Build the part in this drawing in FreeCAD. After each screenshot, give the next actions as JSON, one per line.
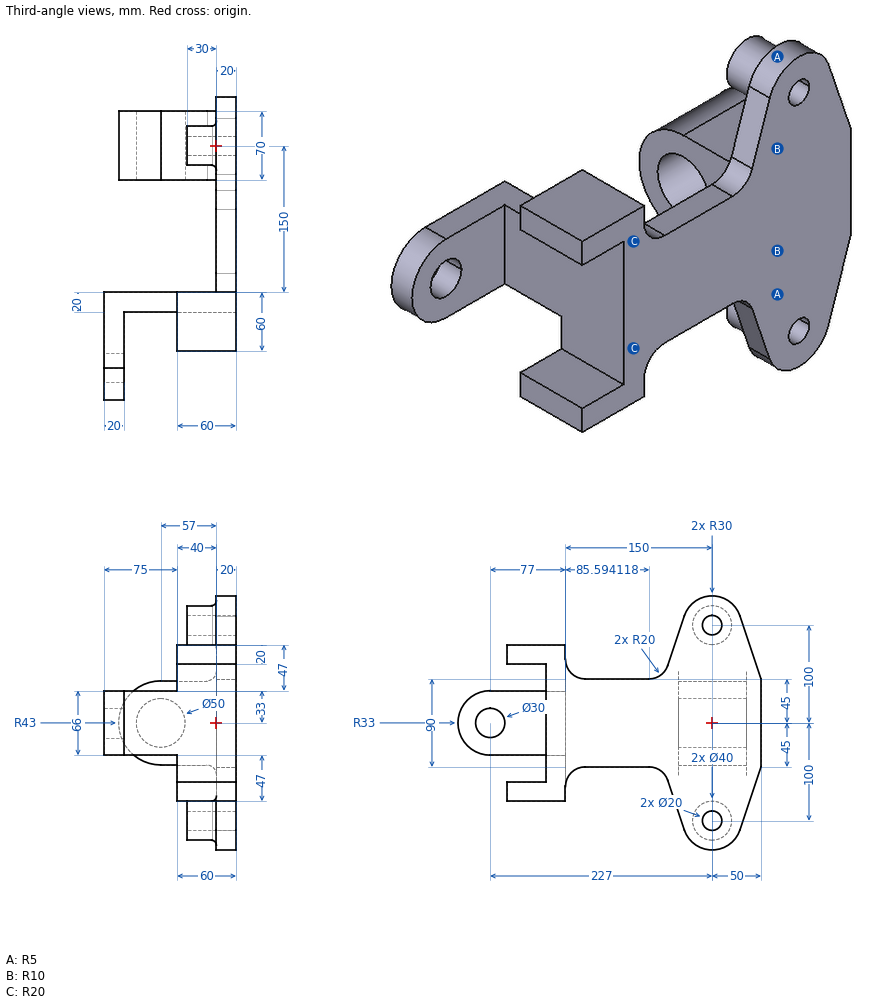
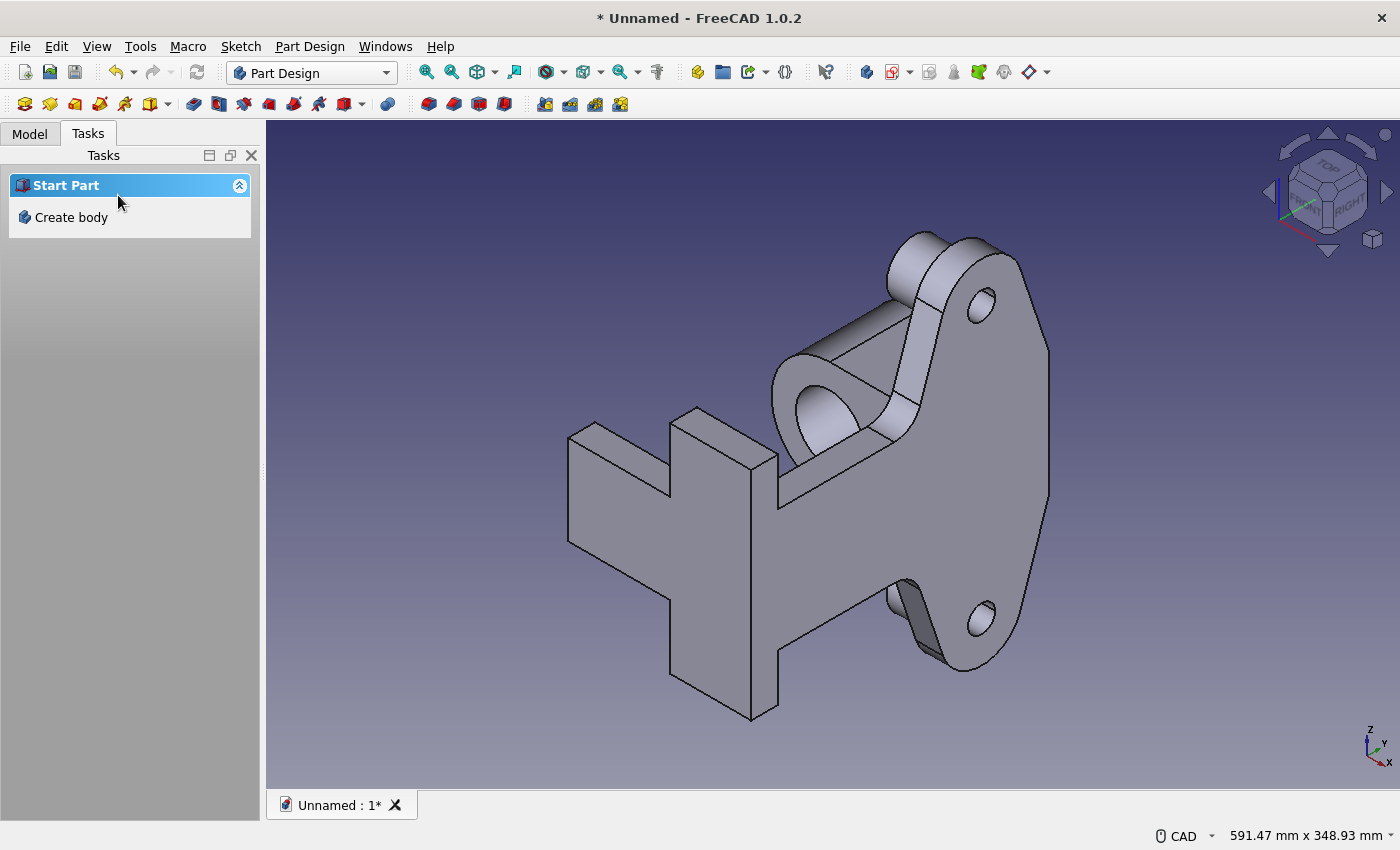
{"action": "key", "text": "v f"}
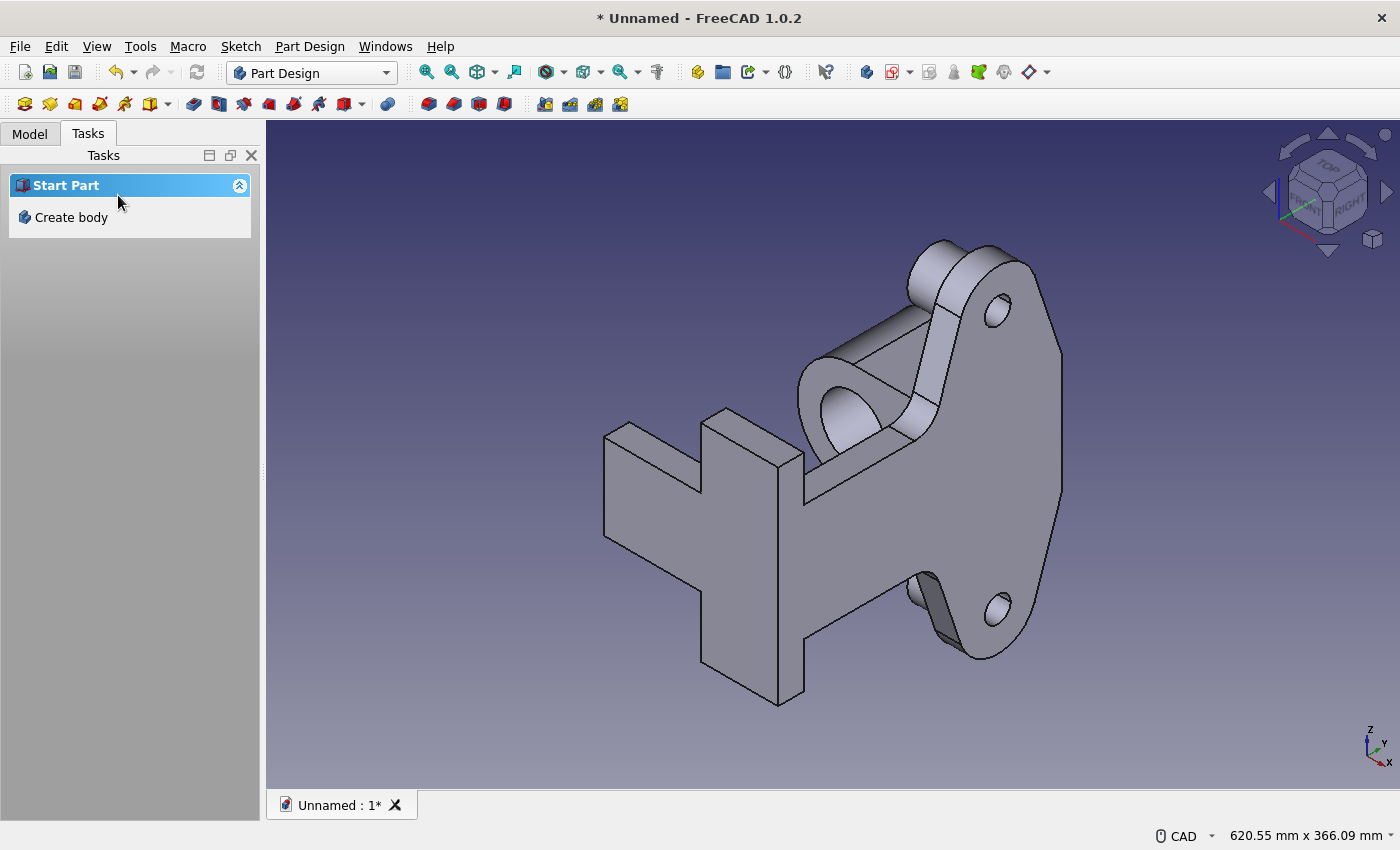
{"action": "key", "text": "6"}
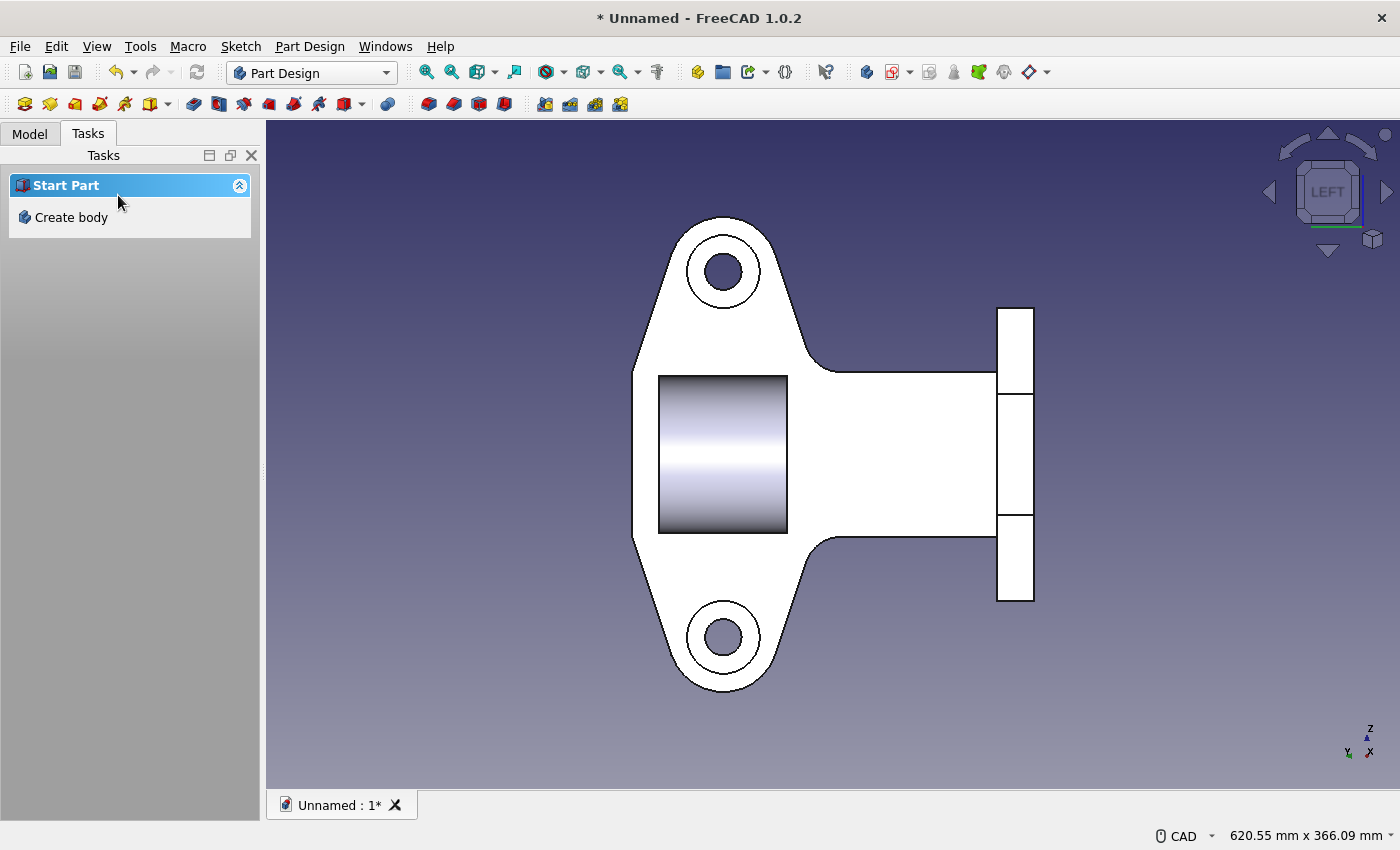
{"action": "left_click", "coordinate": [1016, 436]}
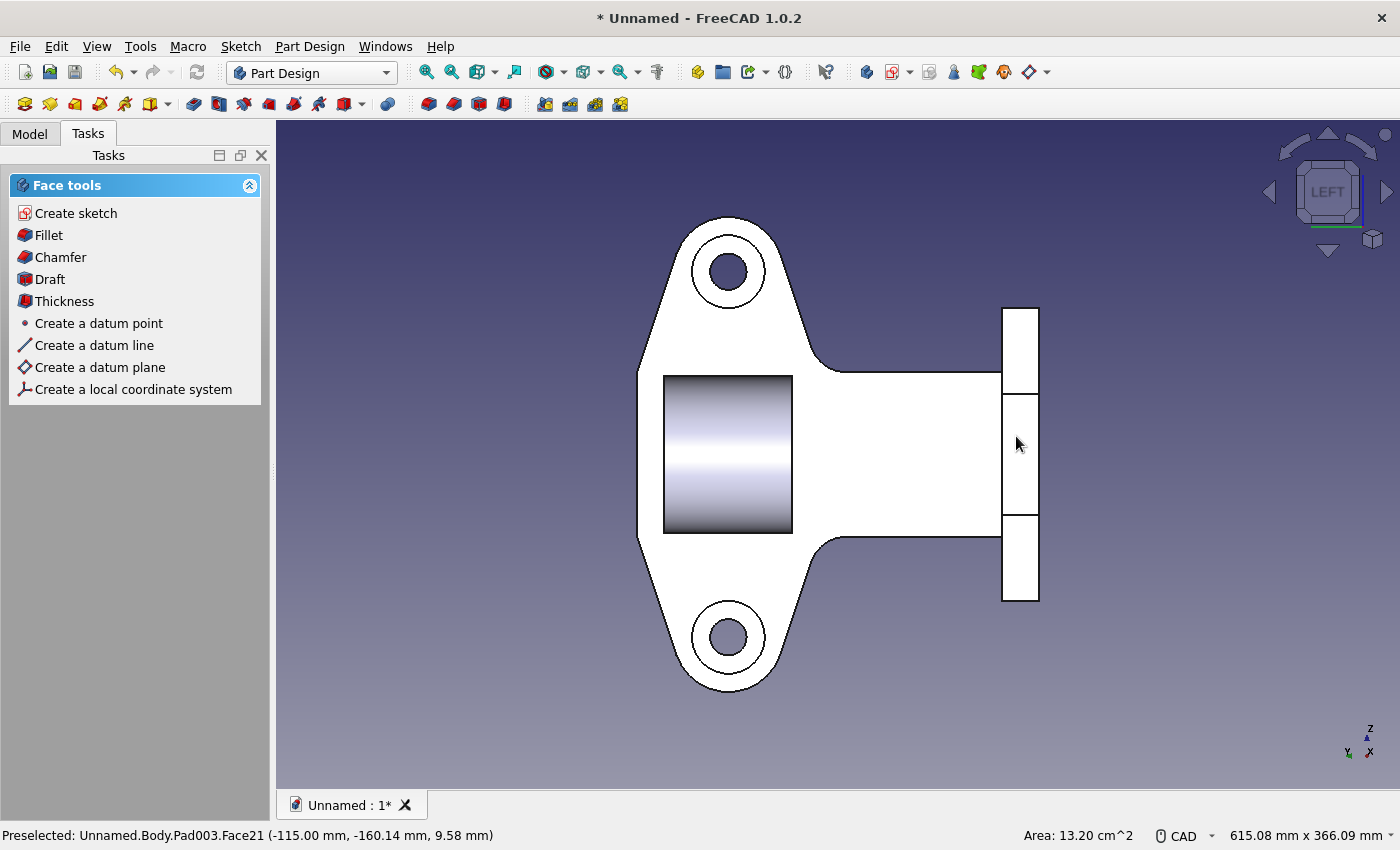
{"action": "left_click", "coordinate": [892, 72]}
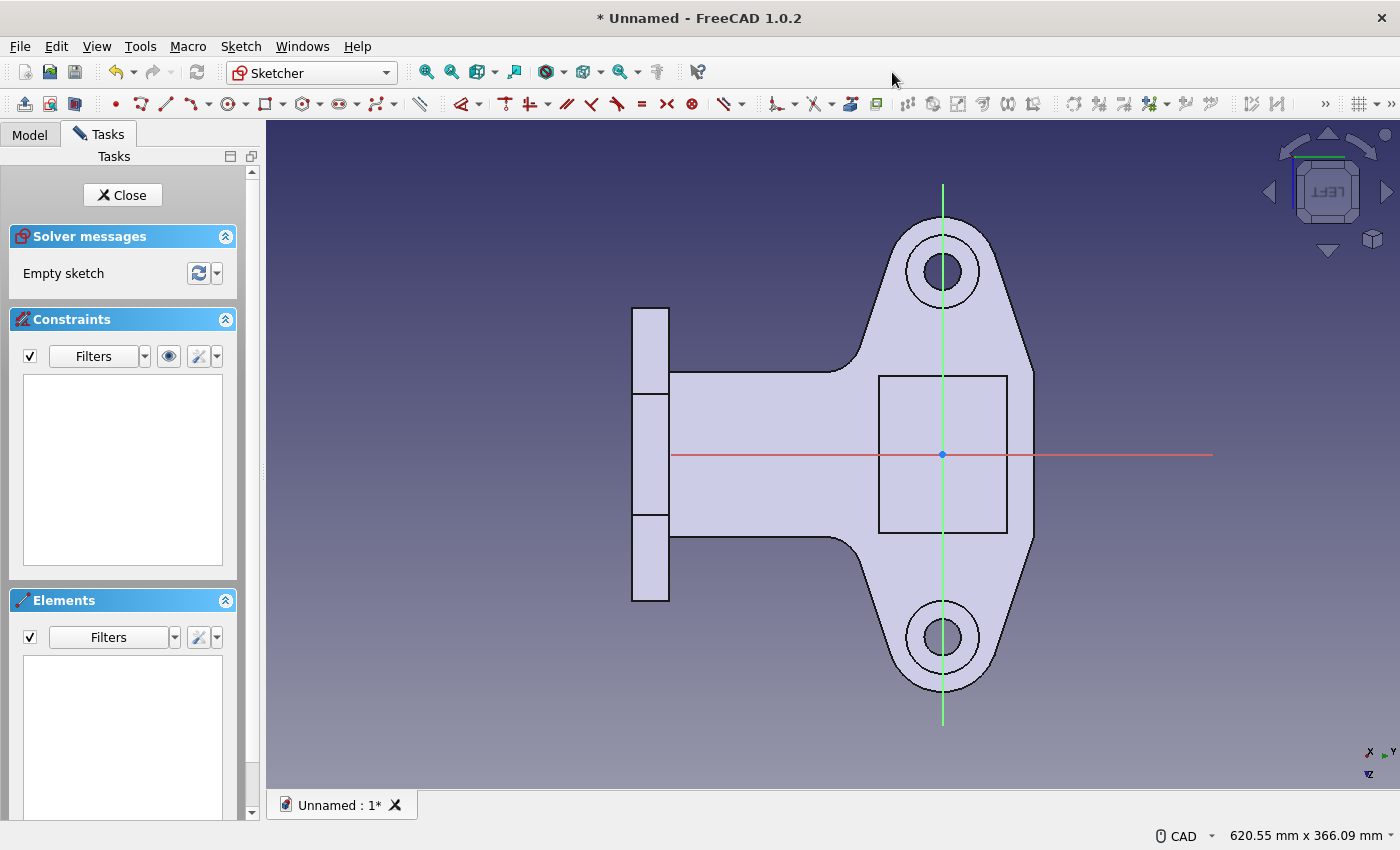
{"action": "scroll", "coordinate": [584, 455], "scroll_direction": "up", "scroll_amount": 2}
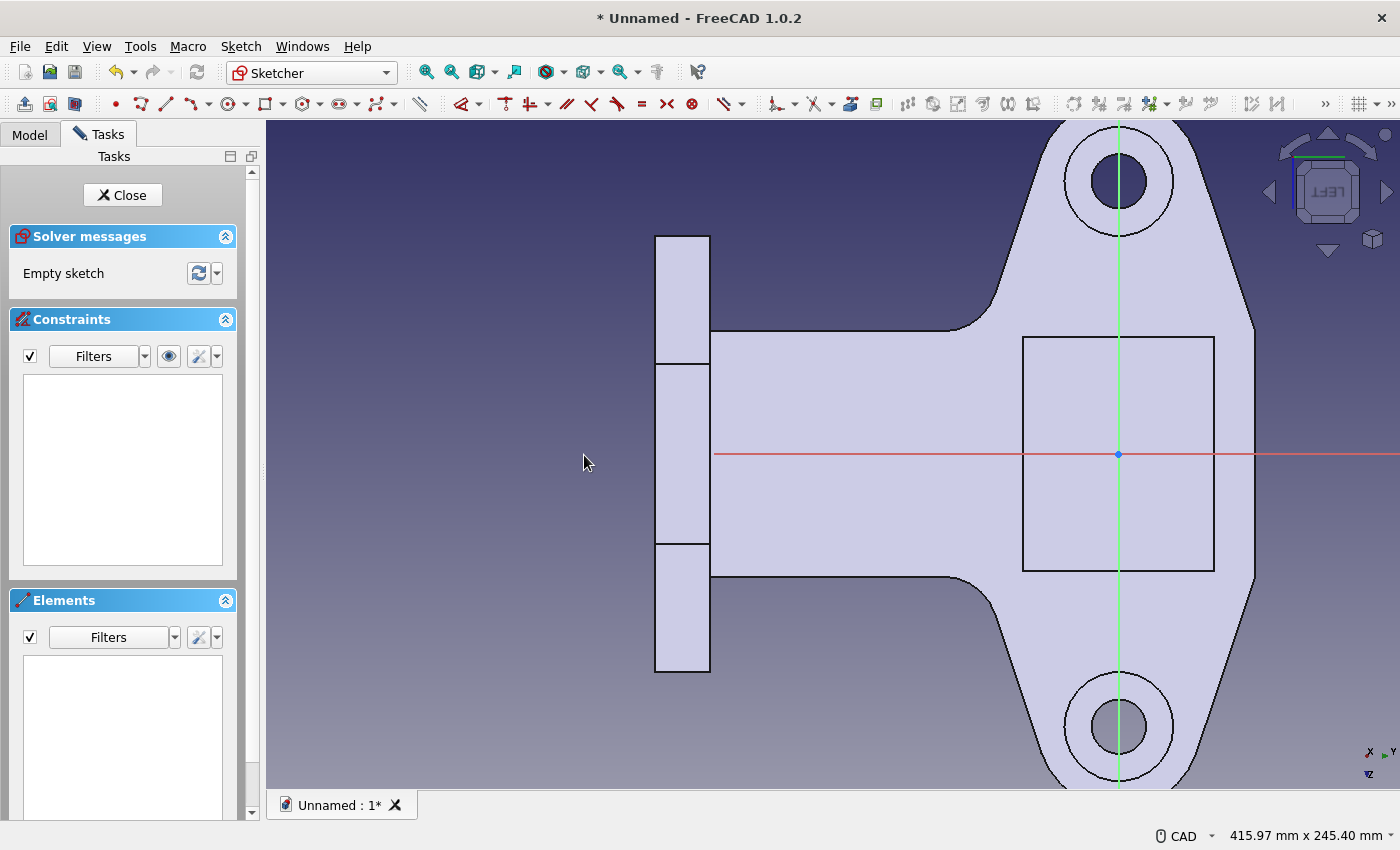
{"action": "left_click", "coordinate": [141, 104]}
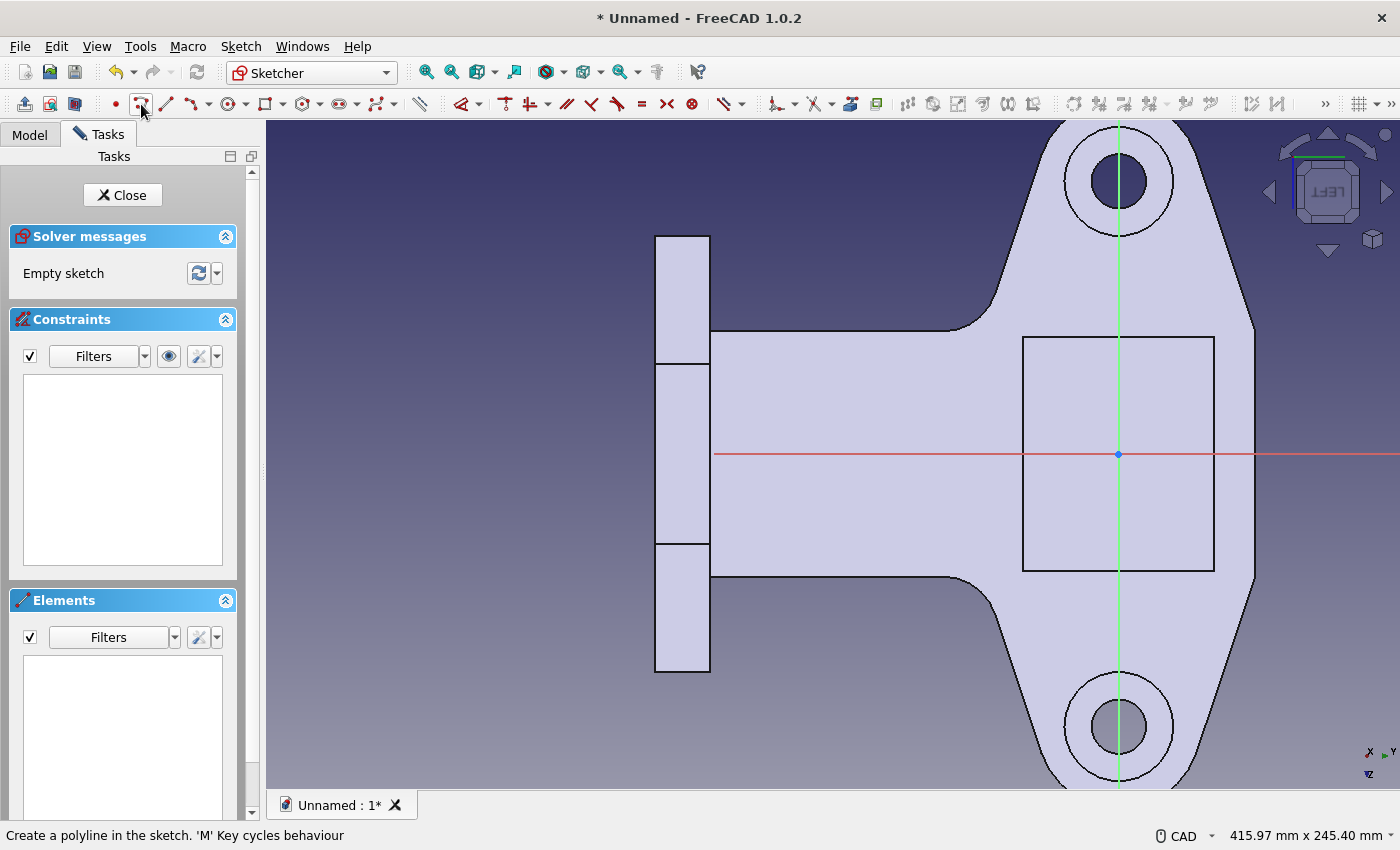
{"action": "left_click", "coordinate": [500, 544]}
{"action": "left_click", "coordinate": [710, 544]}
{"action": "left_click", "coordinate": [710, 364]}
{"action": "left_click", "coordinate": [500, 364]}
{"action": "right_click", "coordinate": [500, 364]}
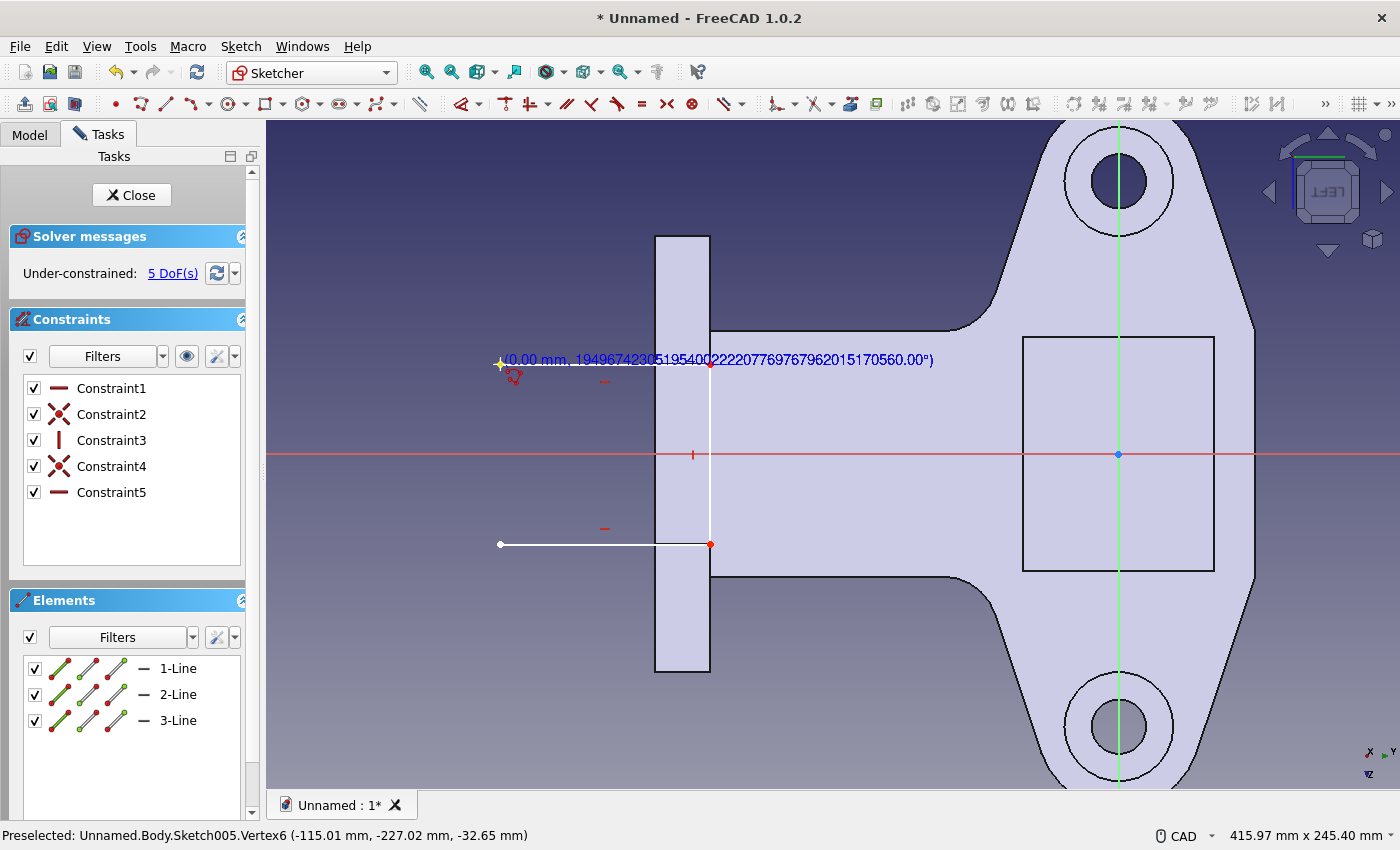
{"action": "left_click", "coordinate": [190, 104]}